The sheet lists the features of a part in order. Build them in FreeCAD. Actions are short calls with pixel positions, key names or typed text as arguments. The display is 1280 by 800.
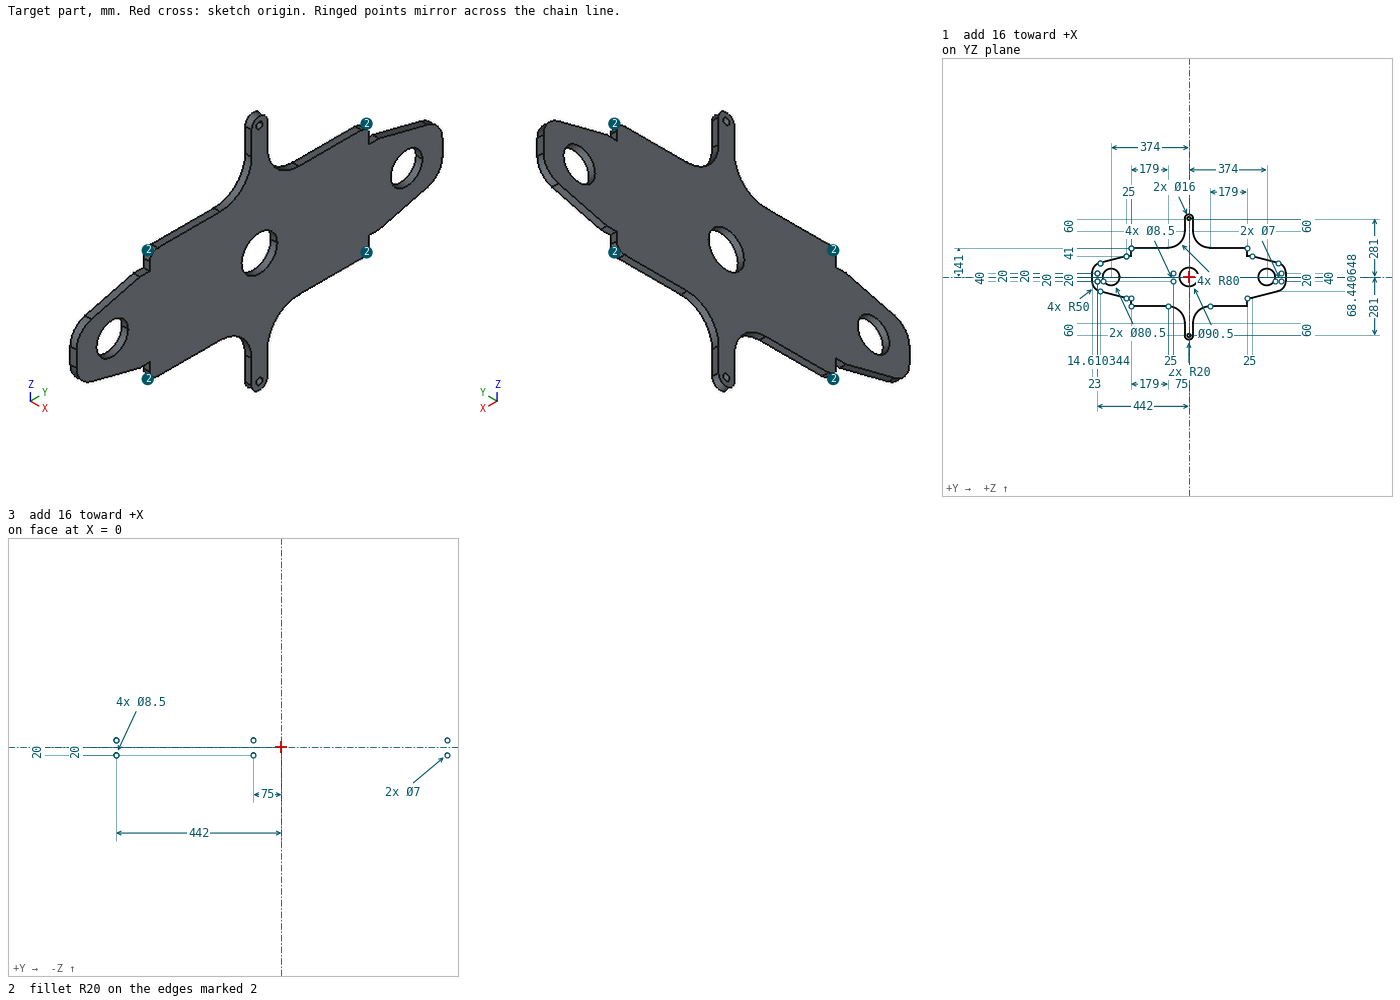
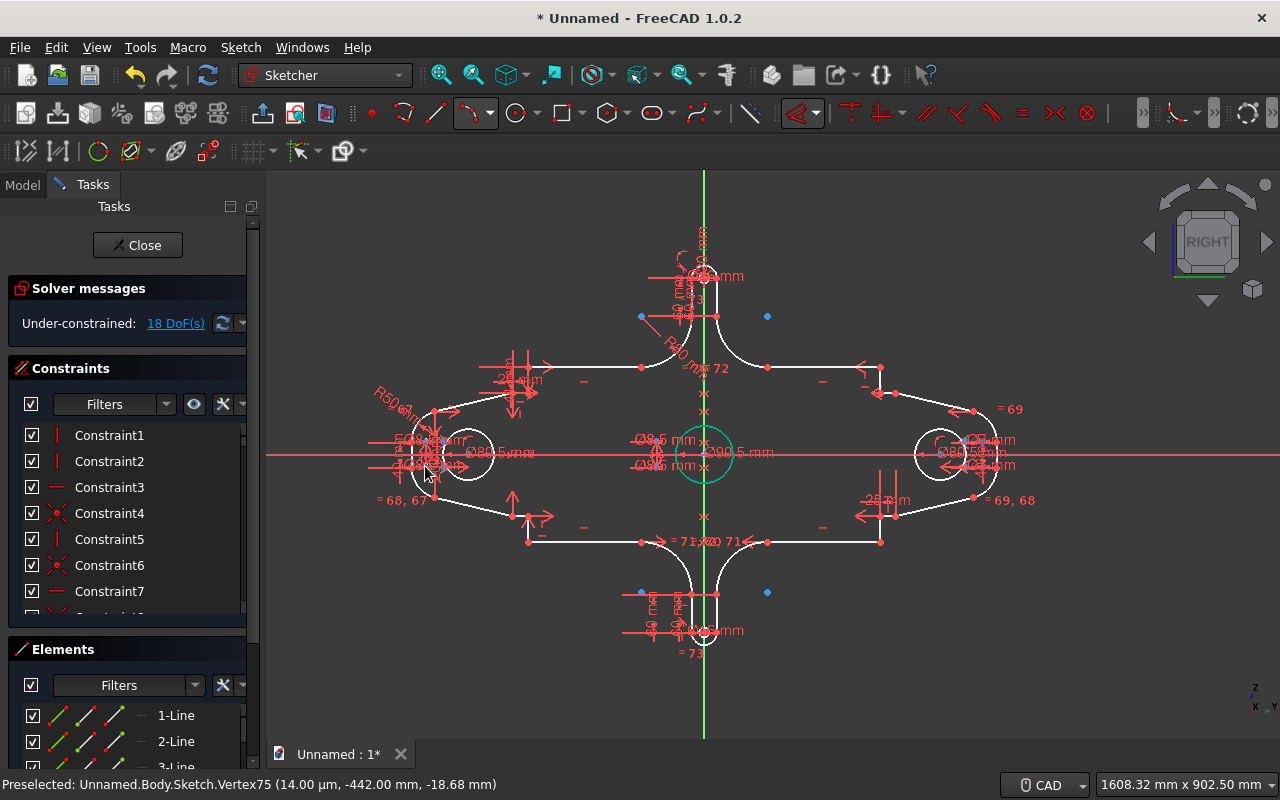
click(657, 468)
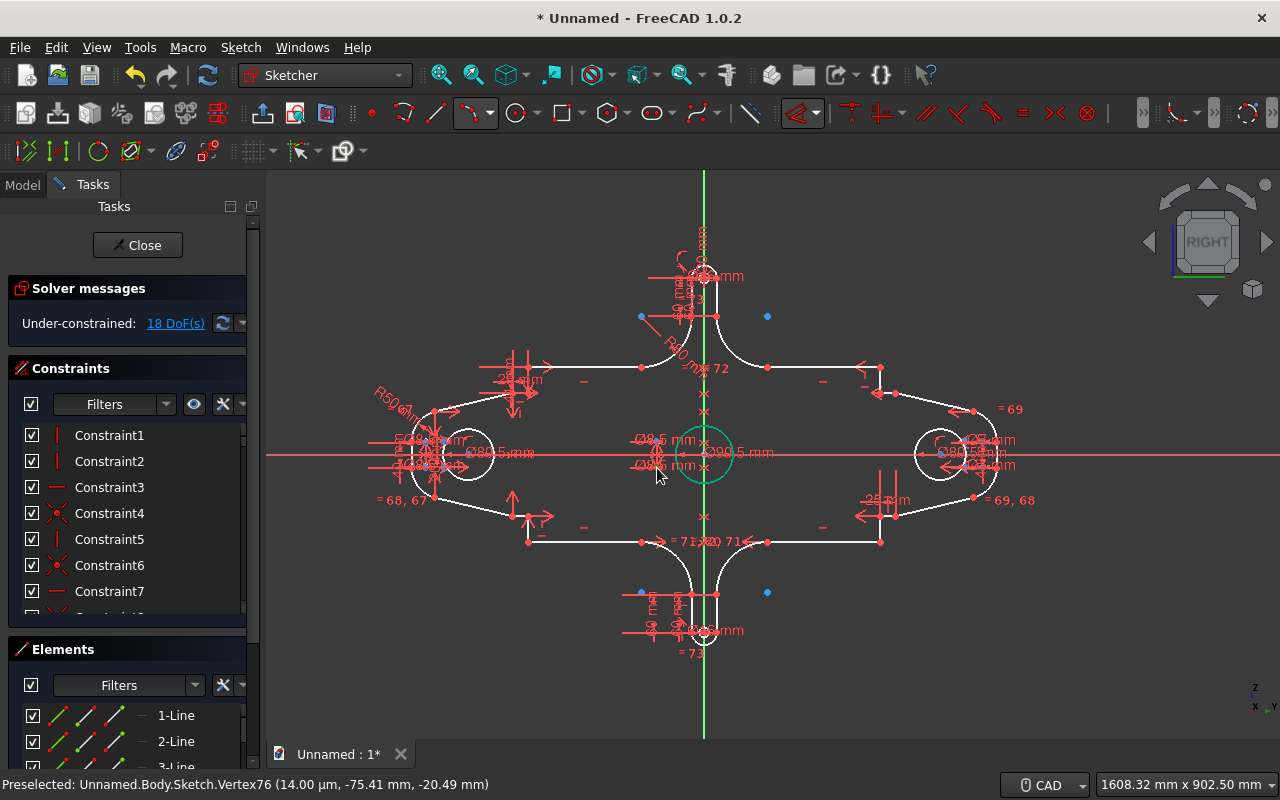
key(l)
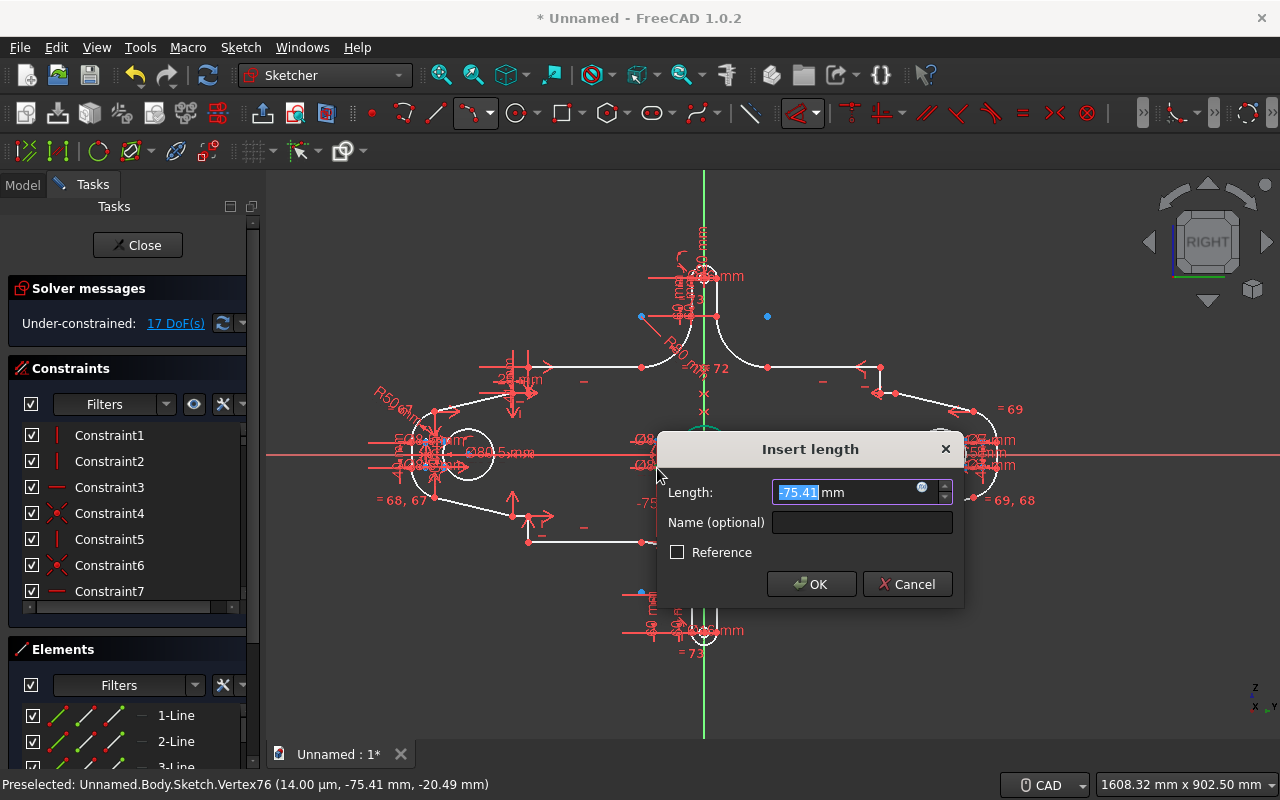
text(-75)
key(Return)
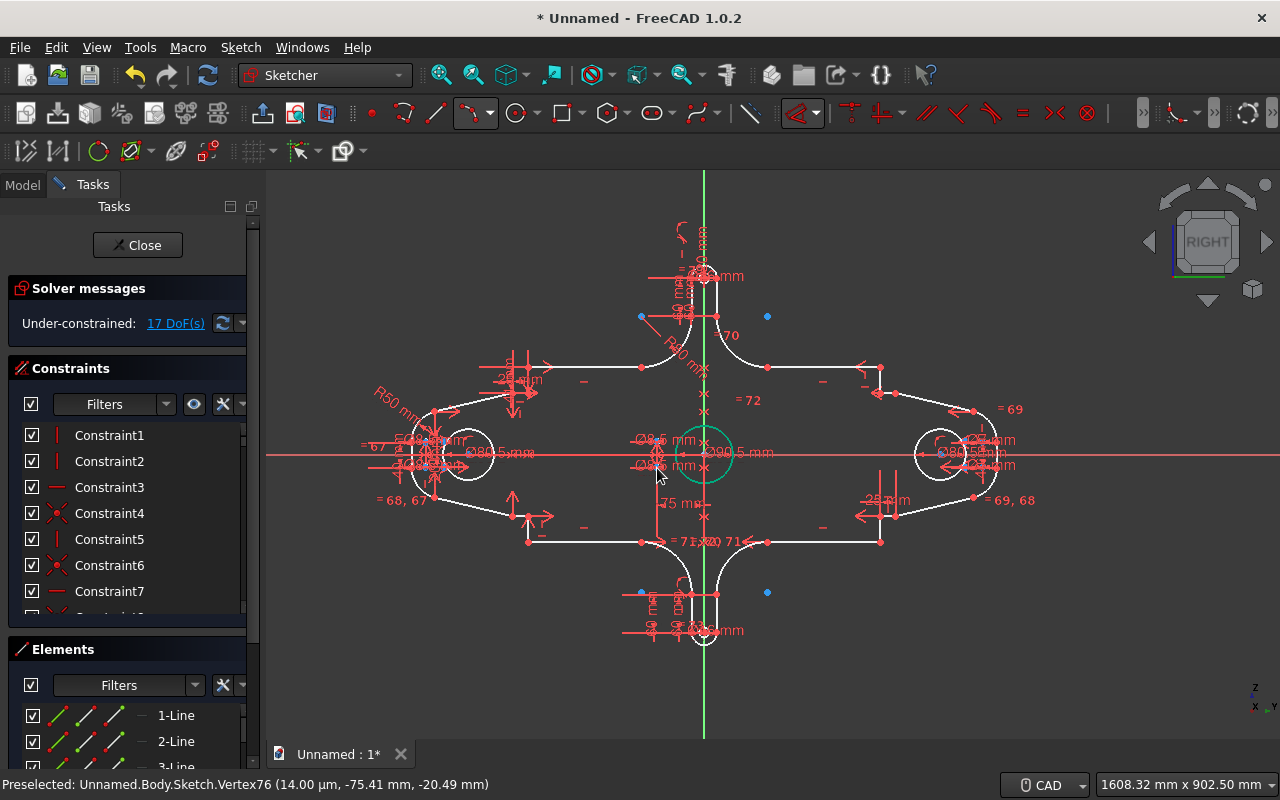
scroll(657, 468, up, 6)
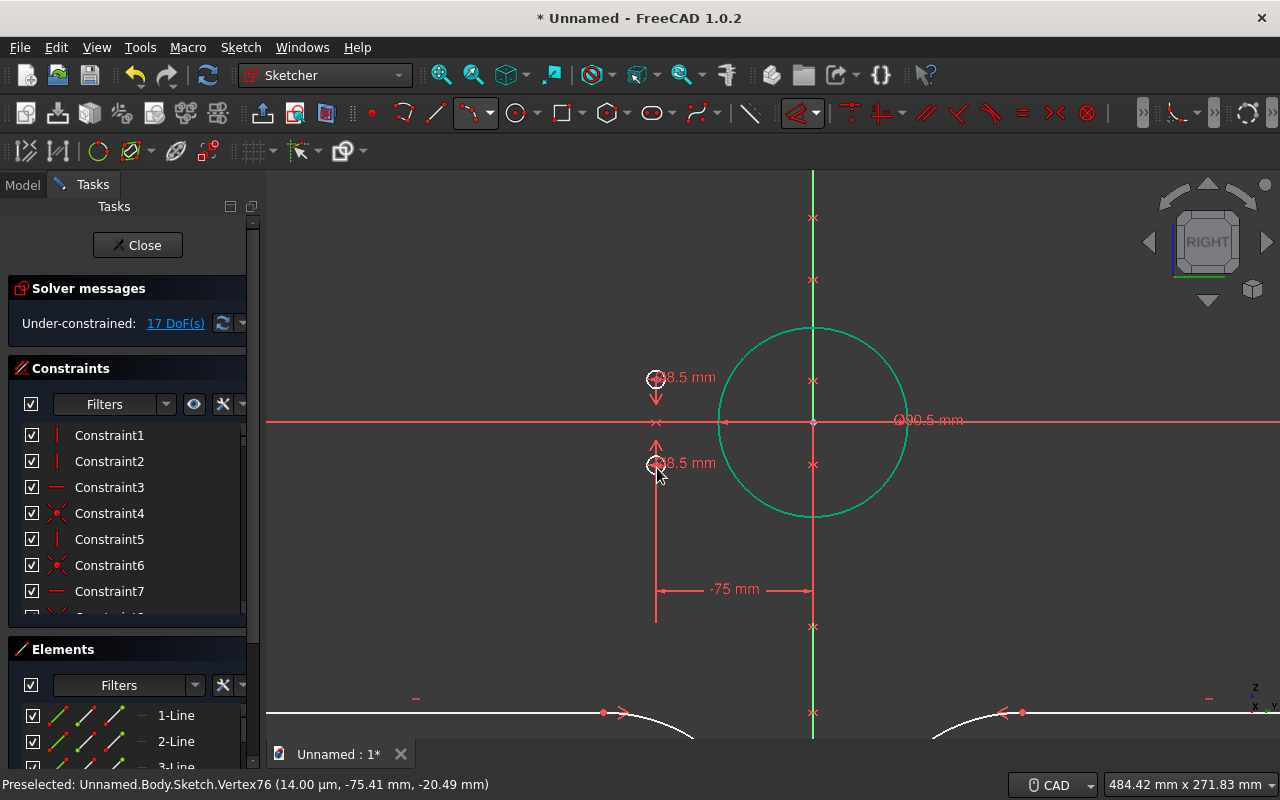
click(656, 465)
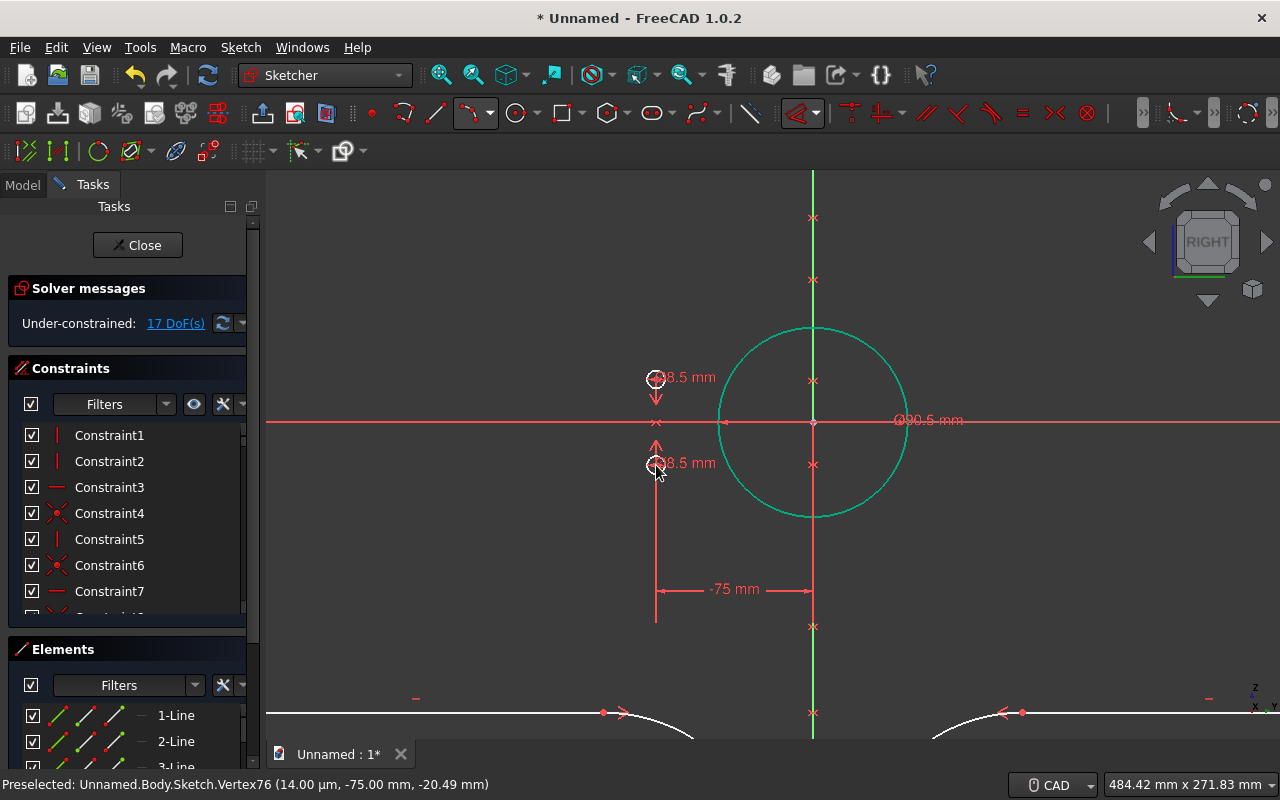
click(818, 114)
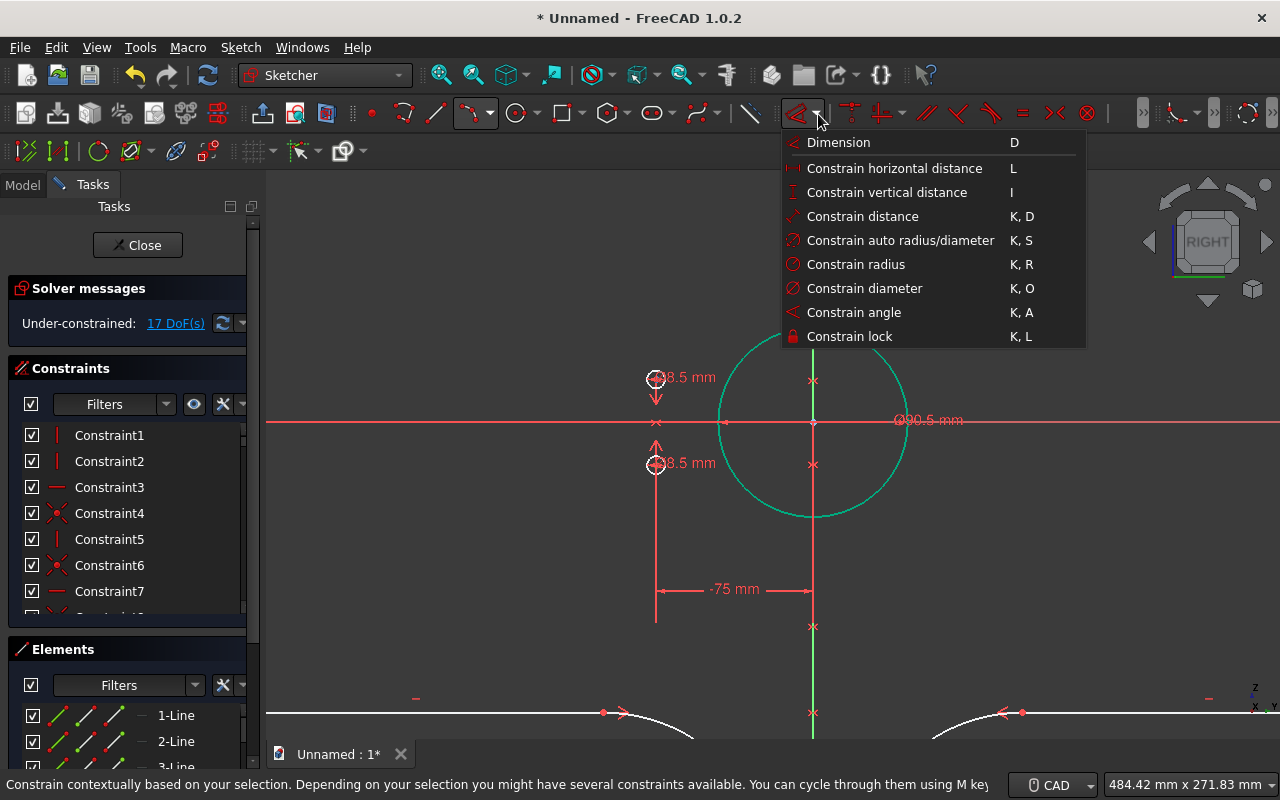
click(934, 192)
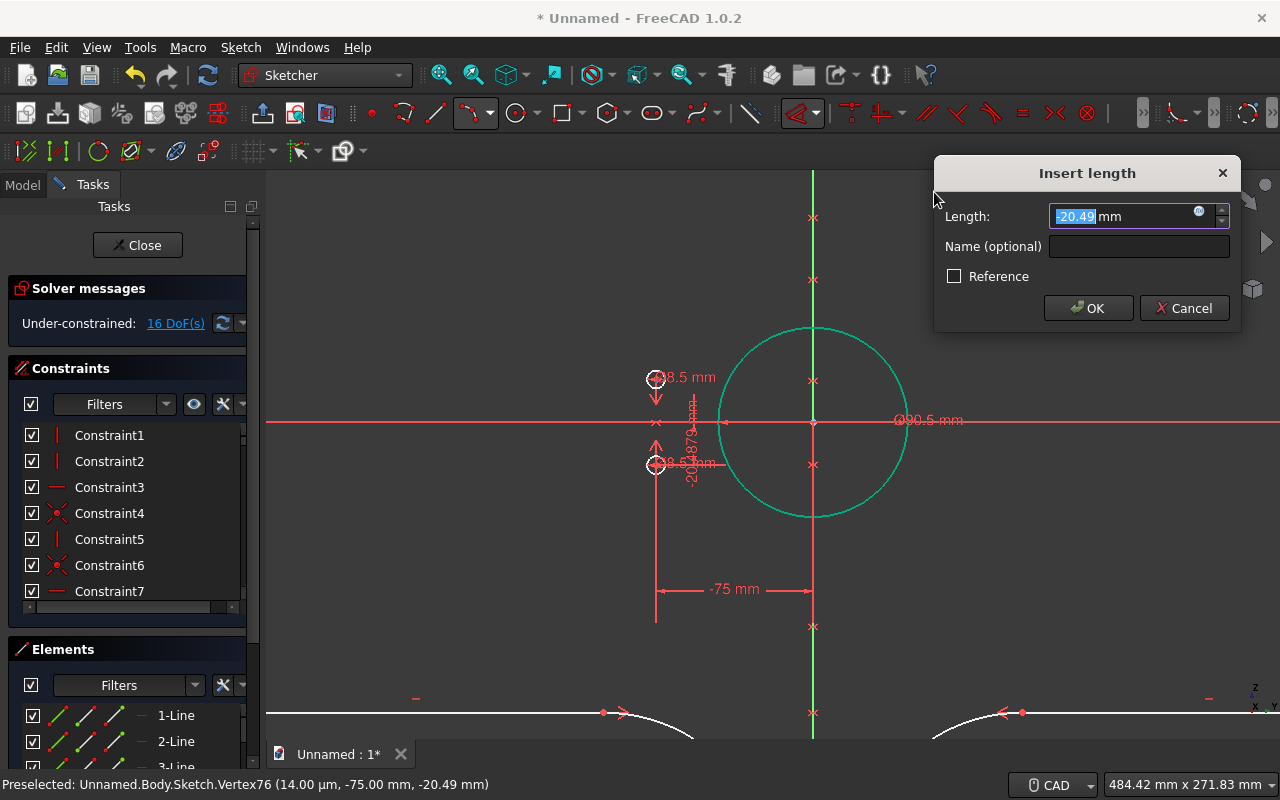
text(-20)
key(Return)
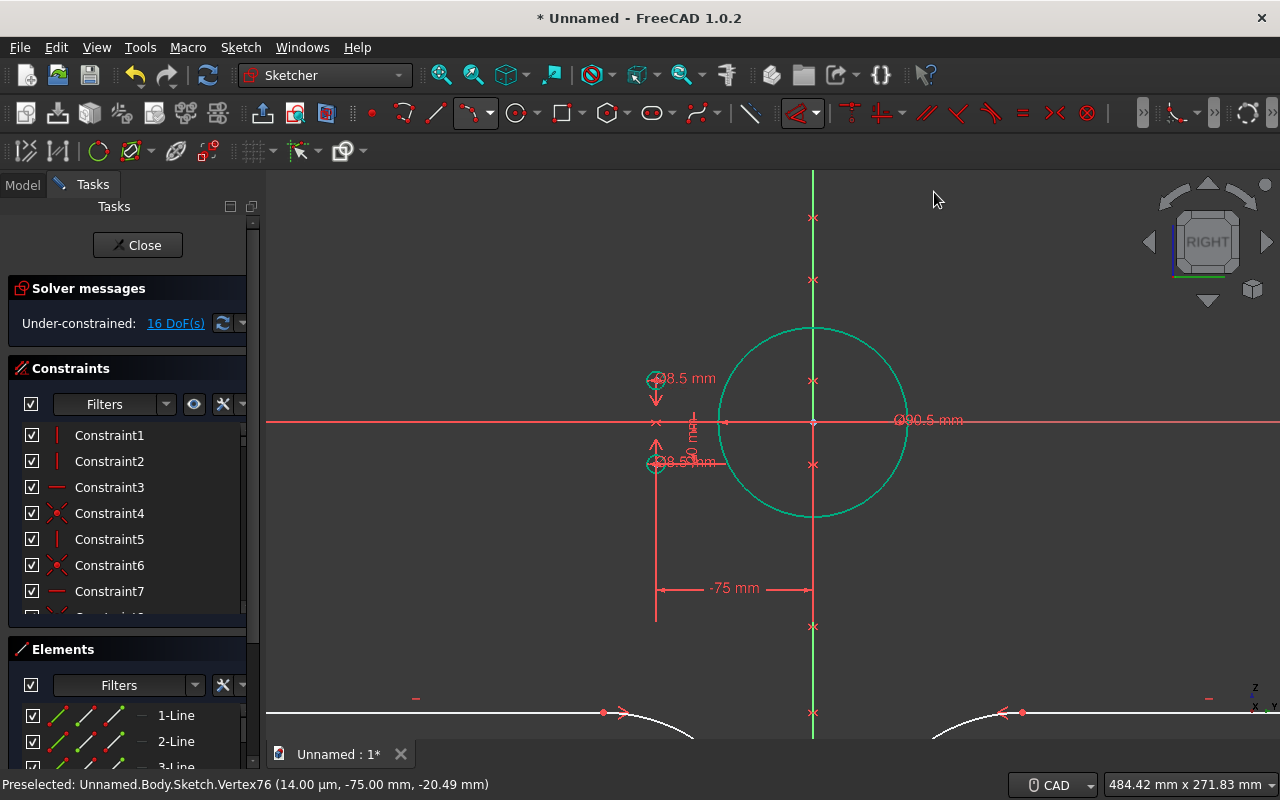
scroll(658, 468, down, 6)